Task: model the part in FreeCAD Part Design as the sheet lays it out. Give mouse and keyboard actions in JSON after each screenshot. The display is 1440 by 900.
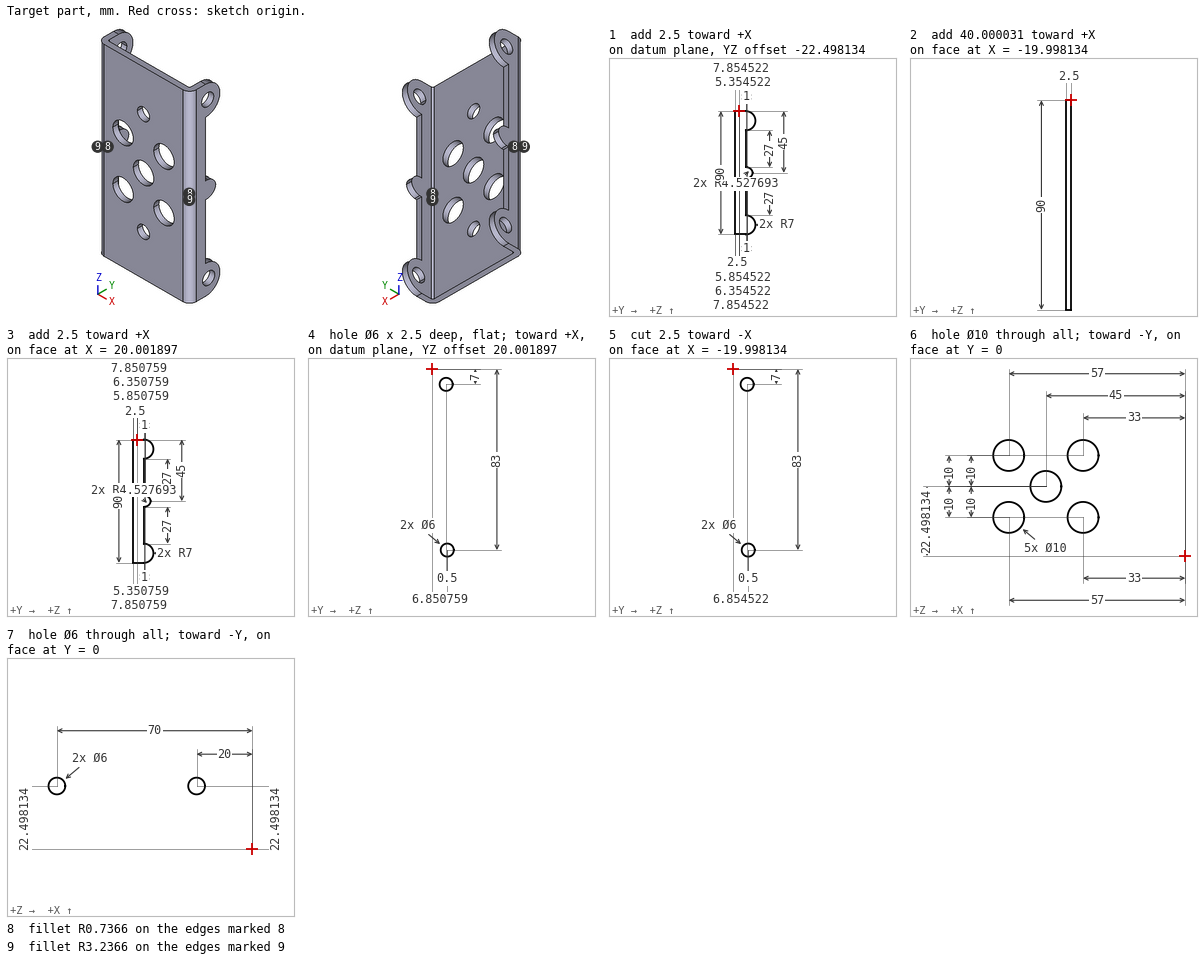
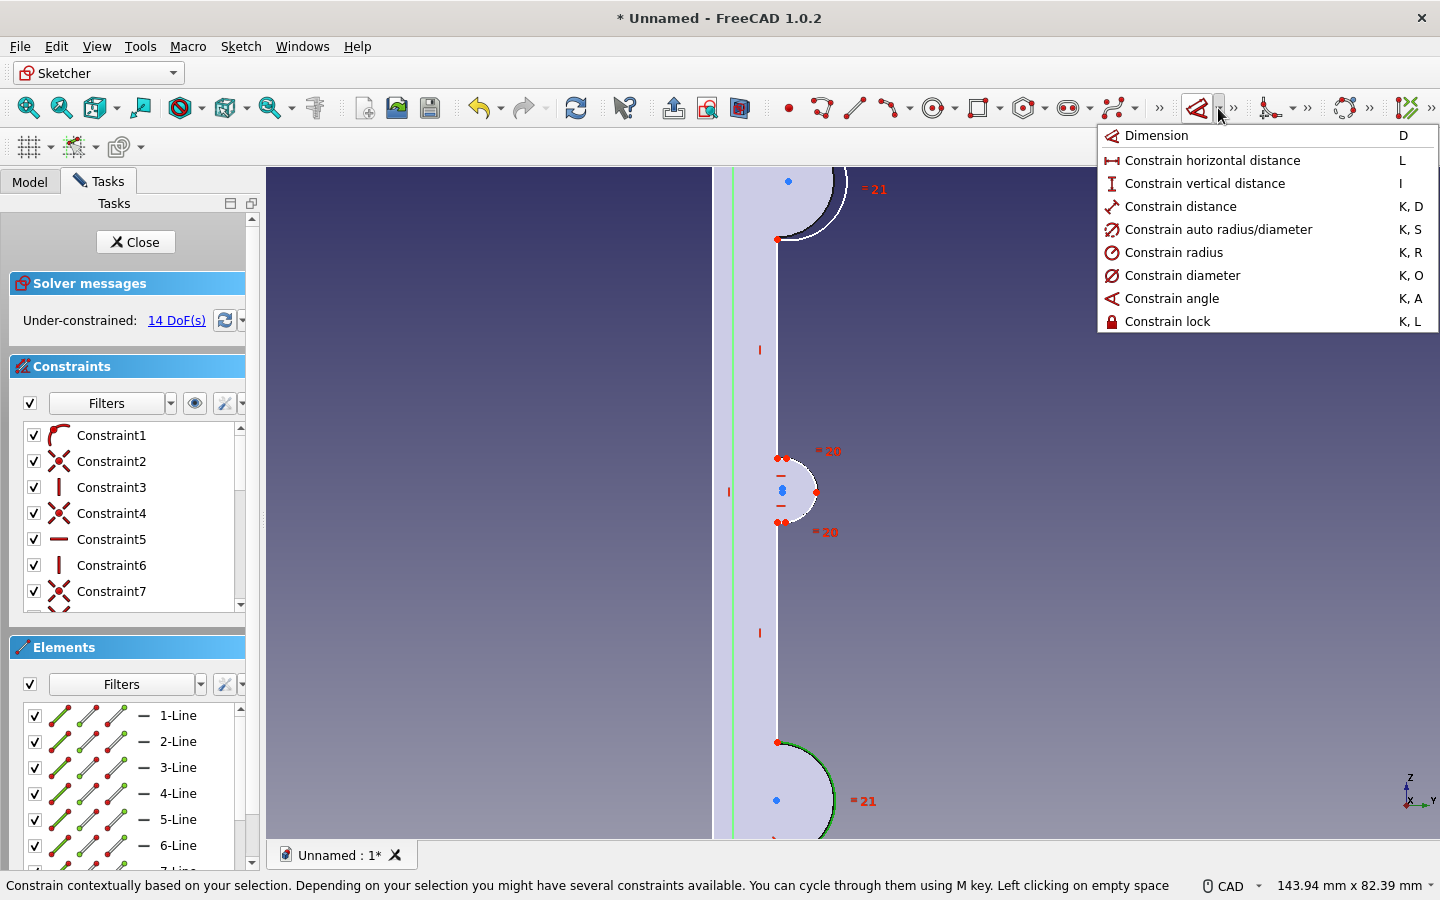
{"action": "left_click", "coordinate": [1268, 252]}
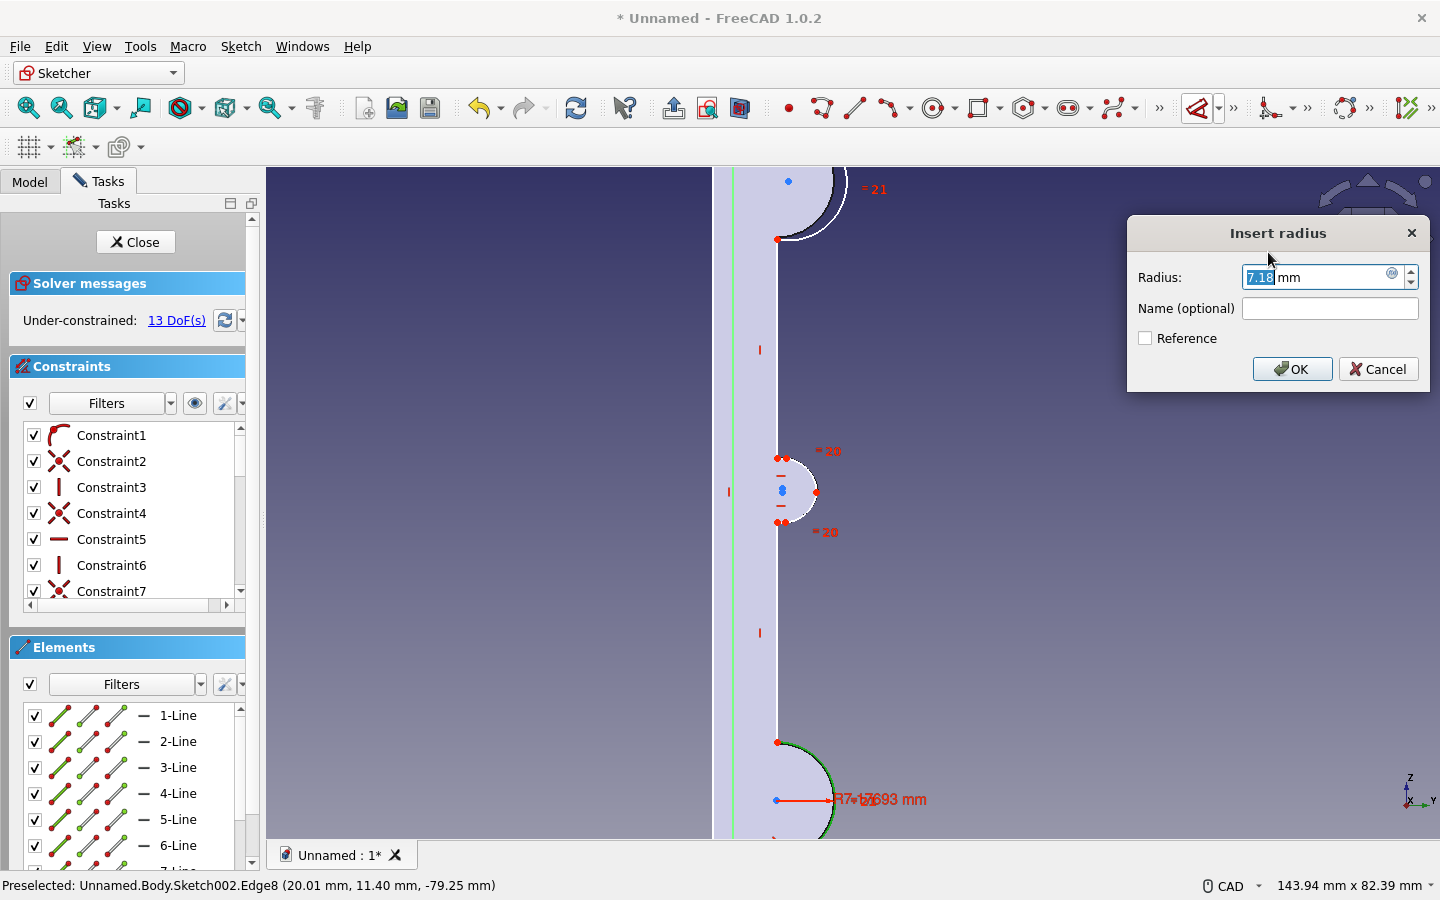
{"action": "type", "text": "7"}
{"action": "key", "text": "Return"}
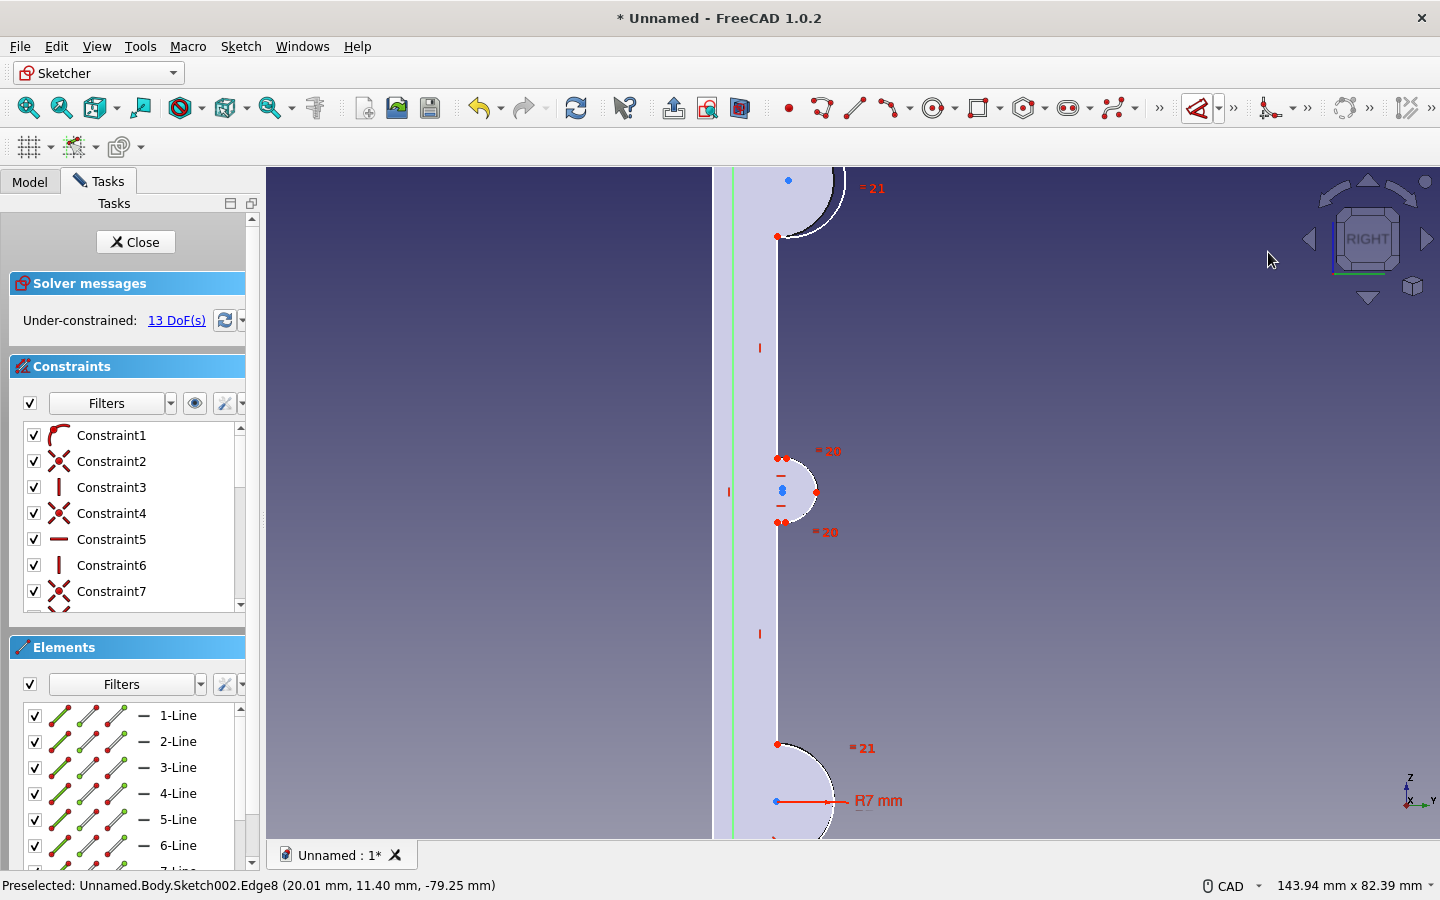
{"action": "left_click", "coordinate": [799, 519]}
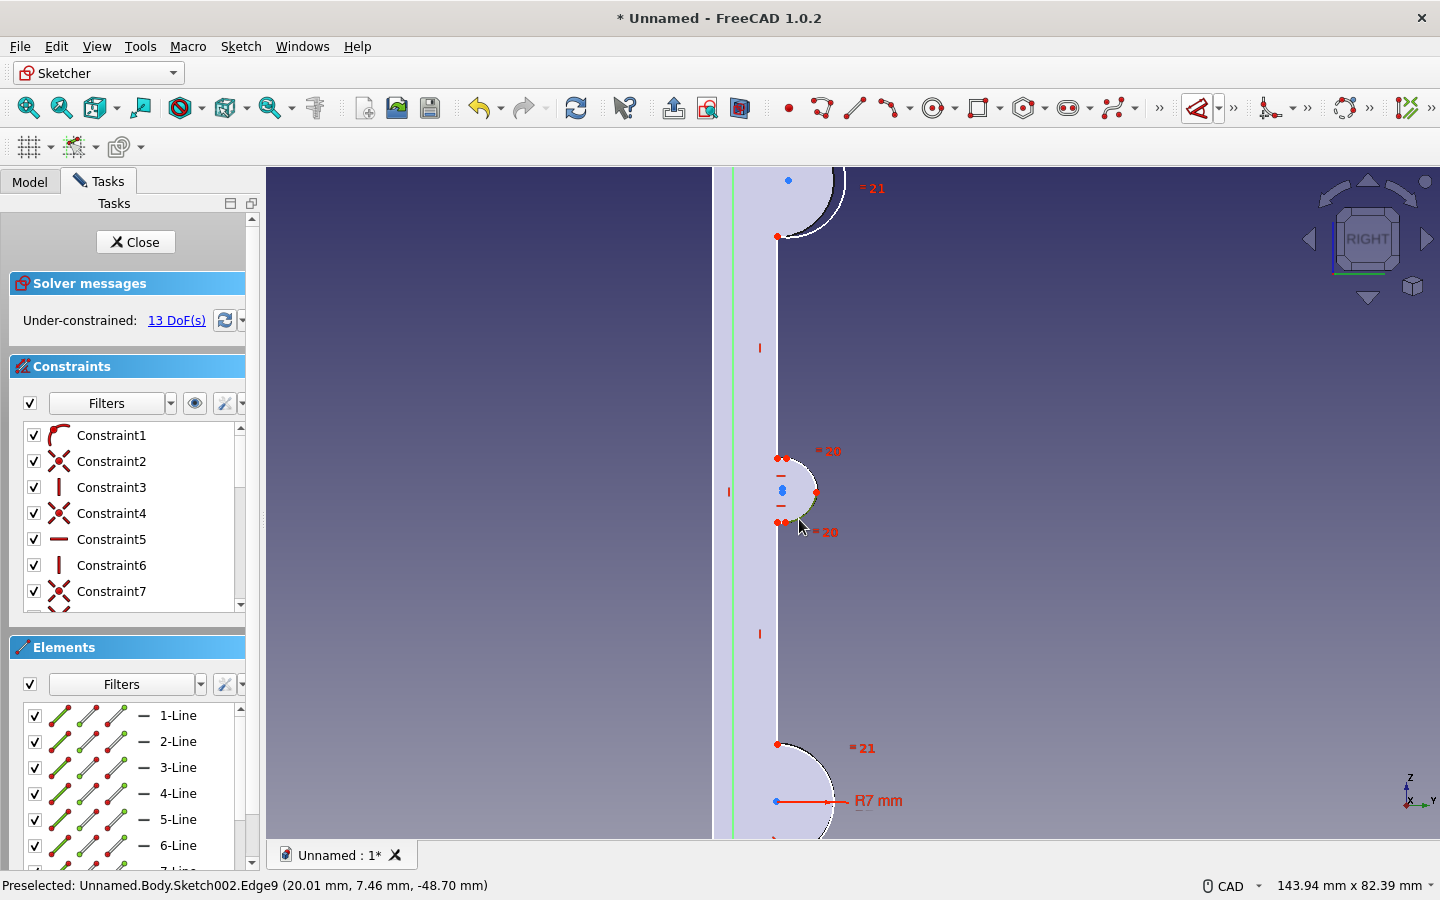
{"action": "key", "text": "k r"}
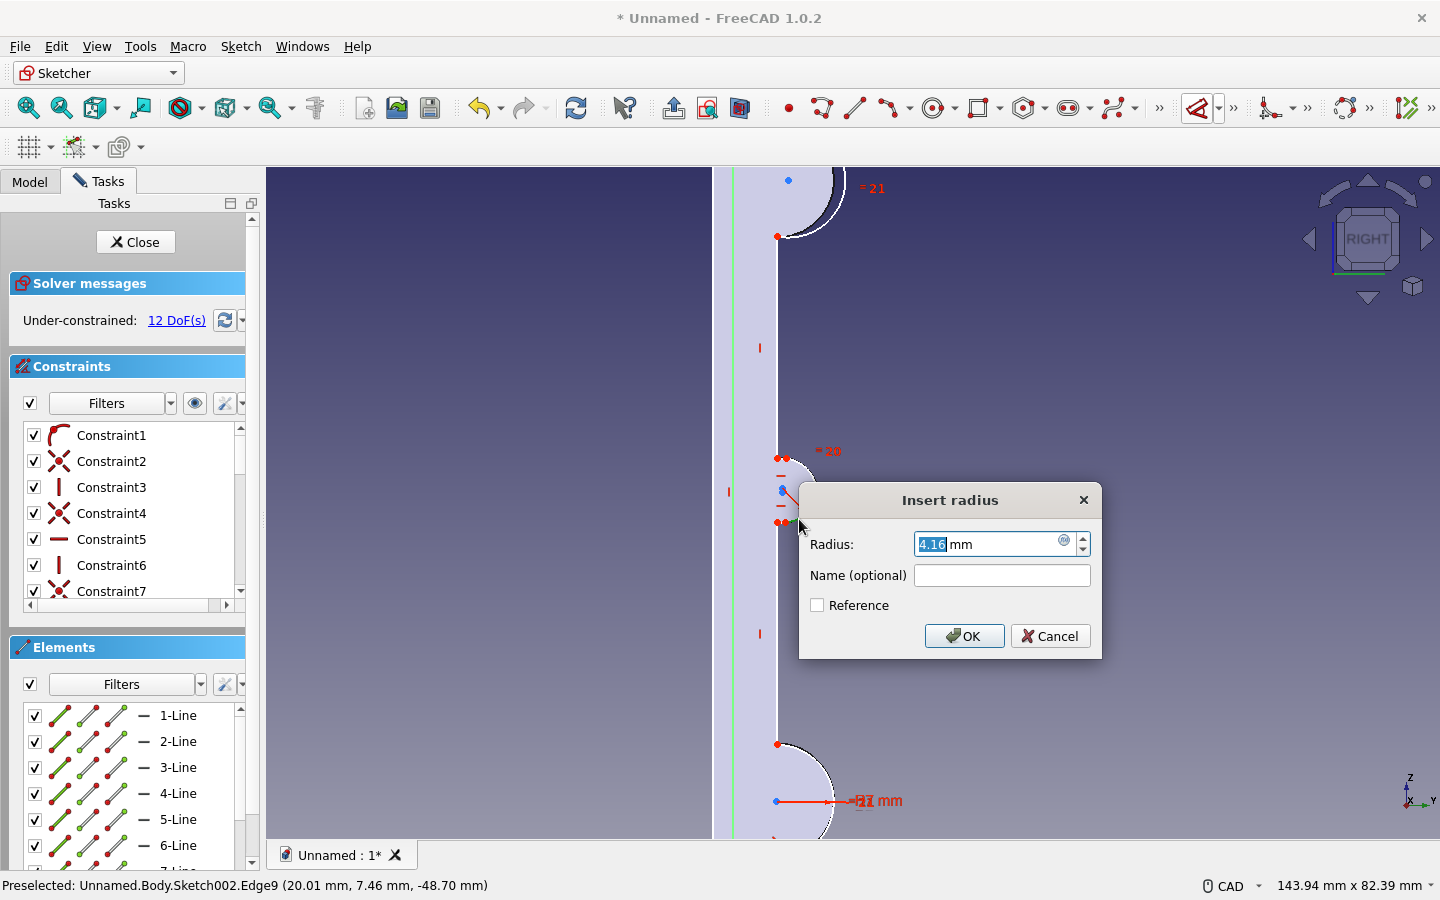
{"action": "type", "text": "4.527693"}
{"action": "key", "text": "Return"}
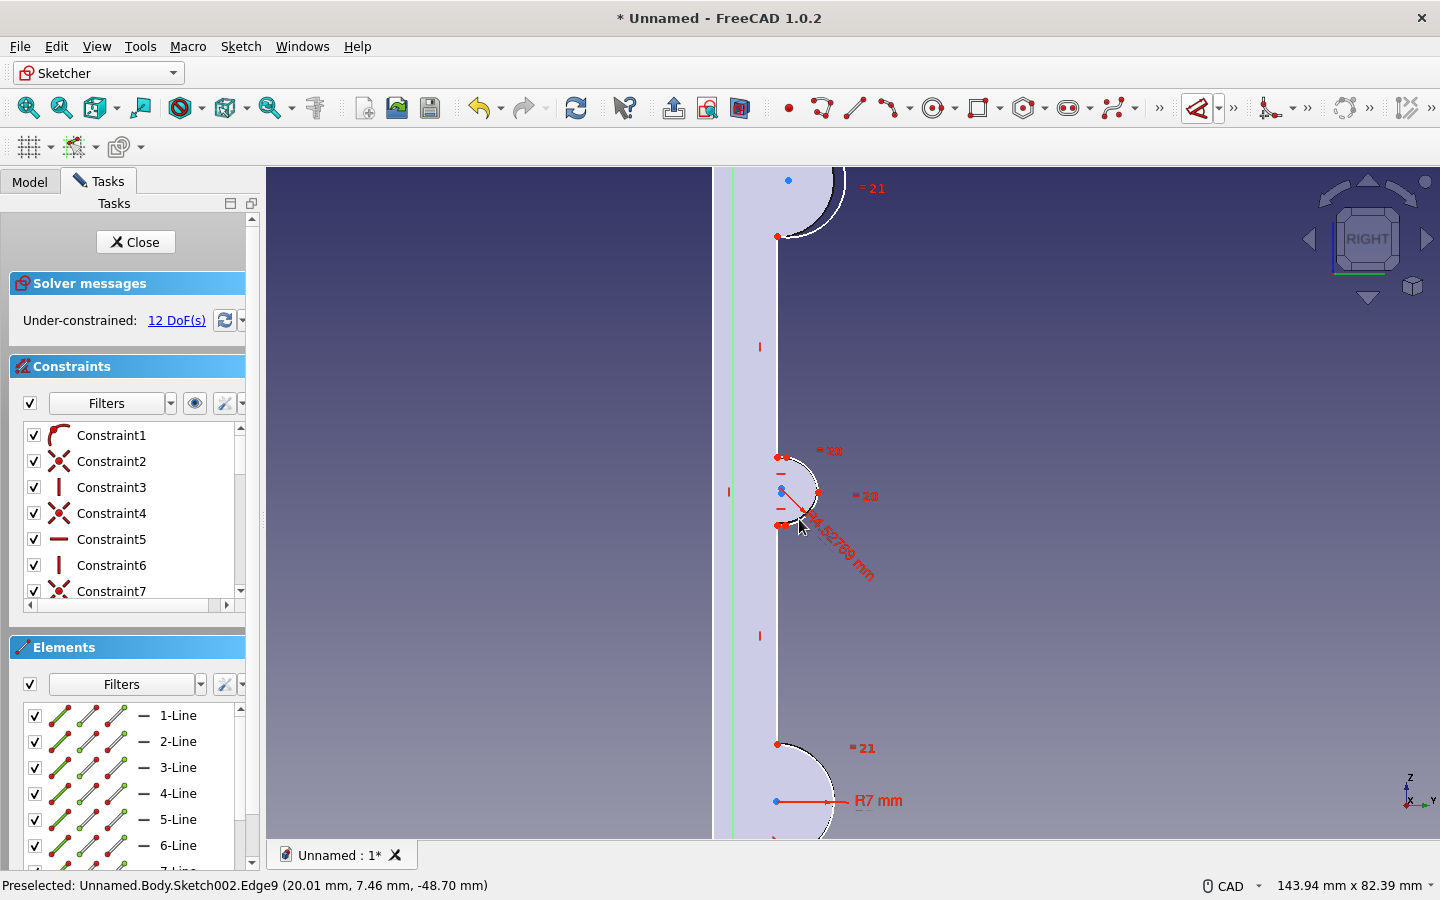
{"action": "scroll", "coordinate": [781, 525], "scroll_direction": "up", "scroll_amount": 8}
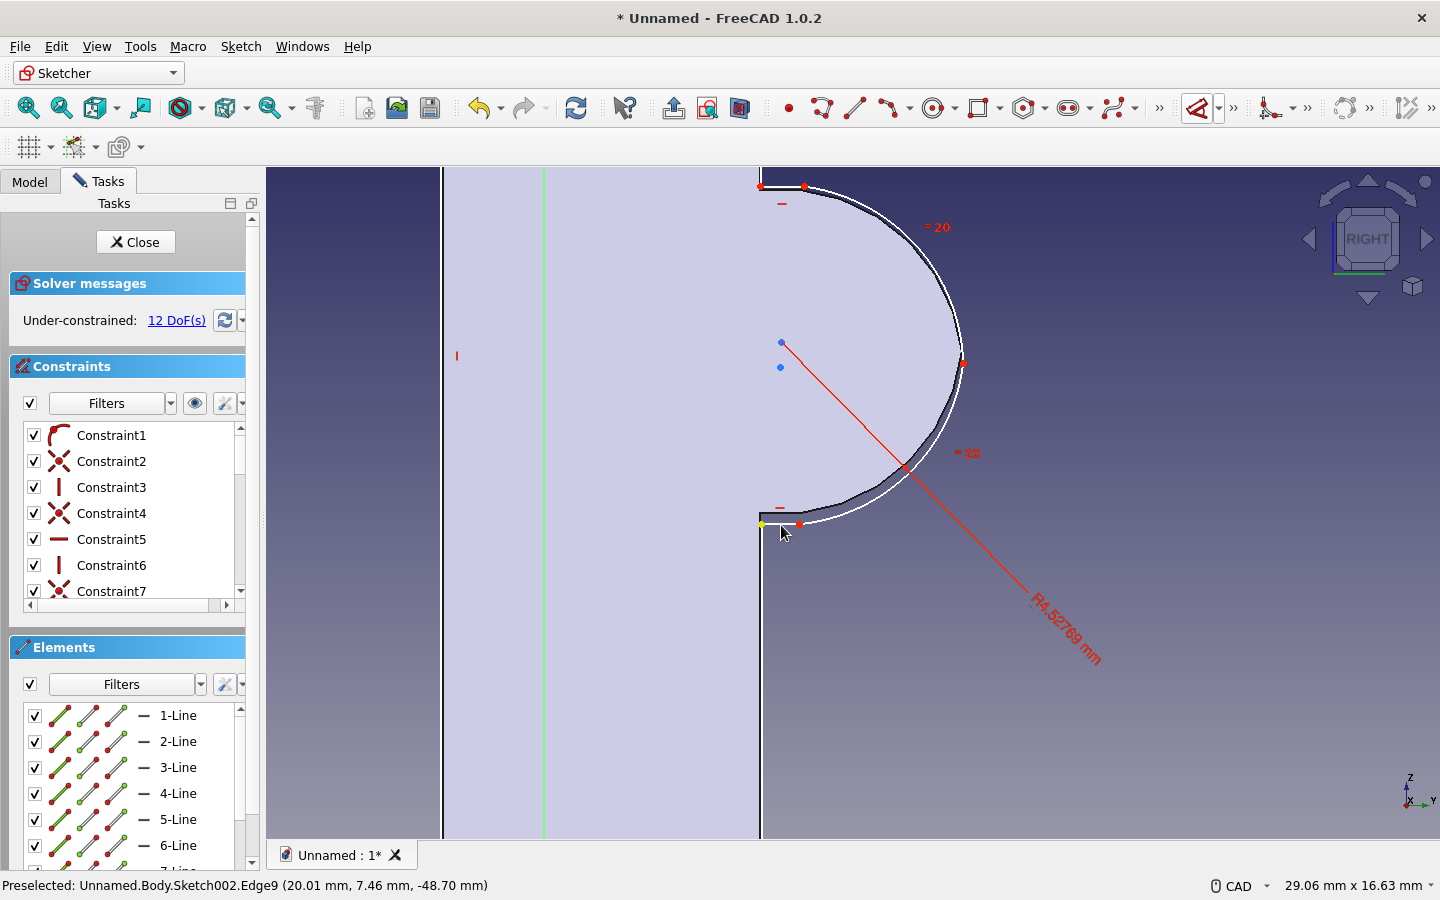
{"action": "left_click", "coordinate": [781, 524]}